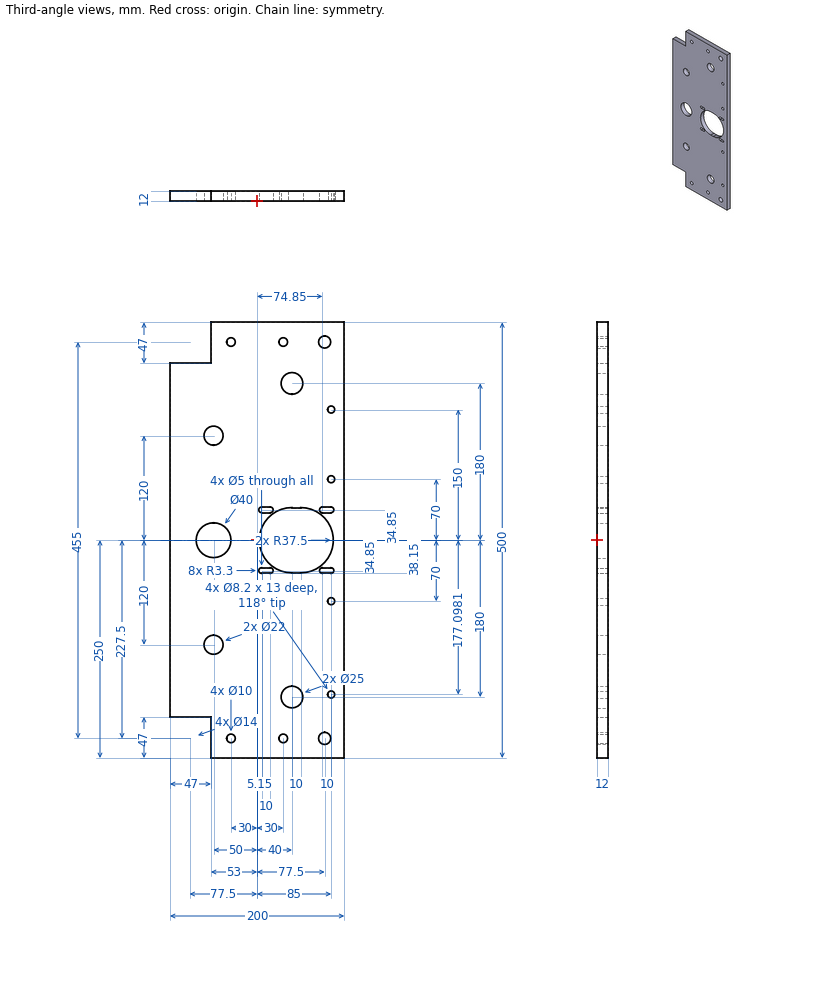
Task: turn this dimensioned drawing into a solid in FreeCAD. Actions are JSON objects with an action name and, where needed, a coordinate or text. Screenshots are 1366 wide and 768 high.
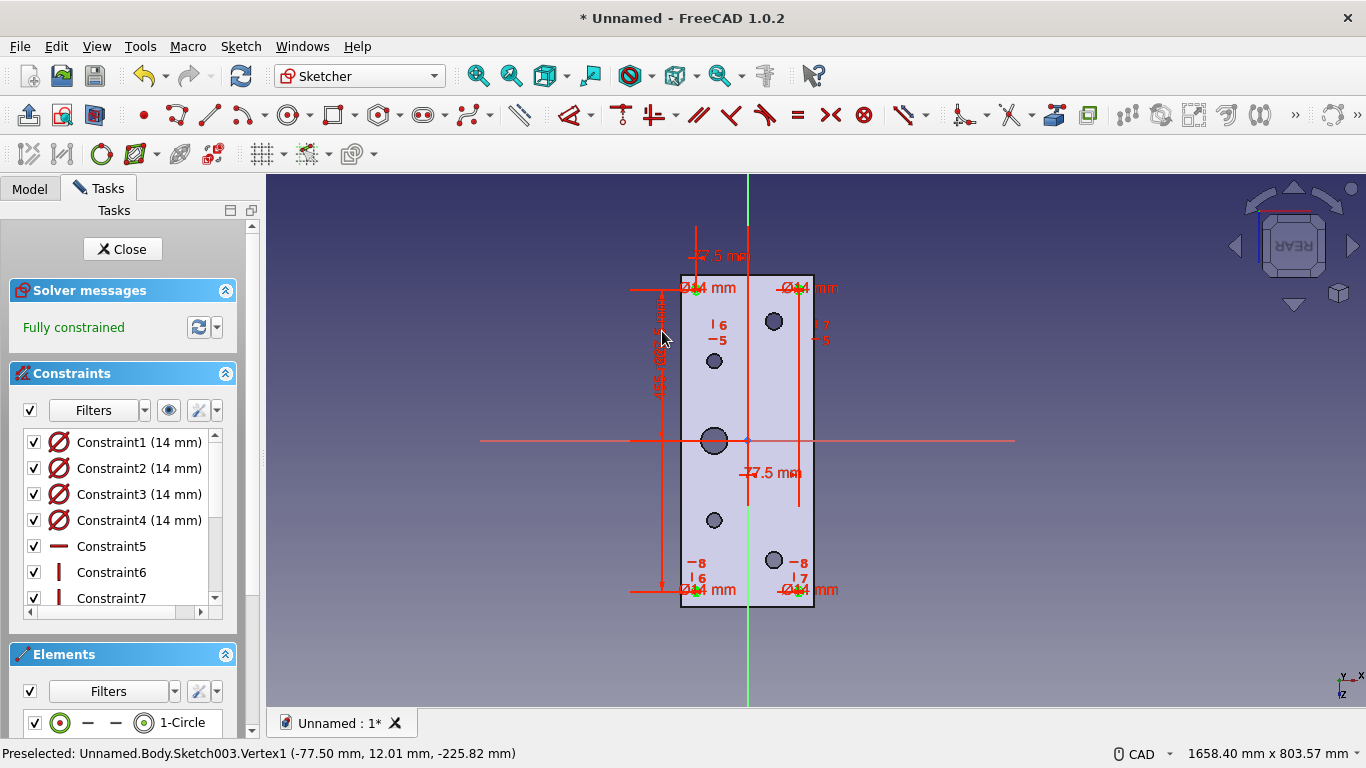
{"action": "left_click", "coordinate": [123, 249]}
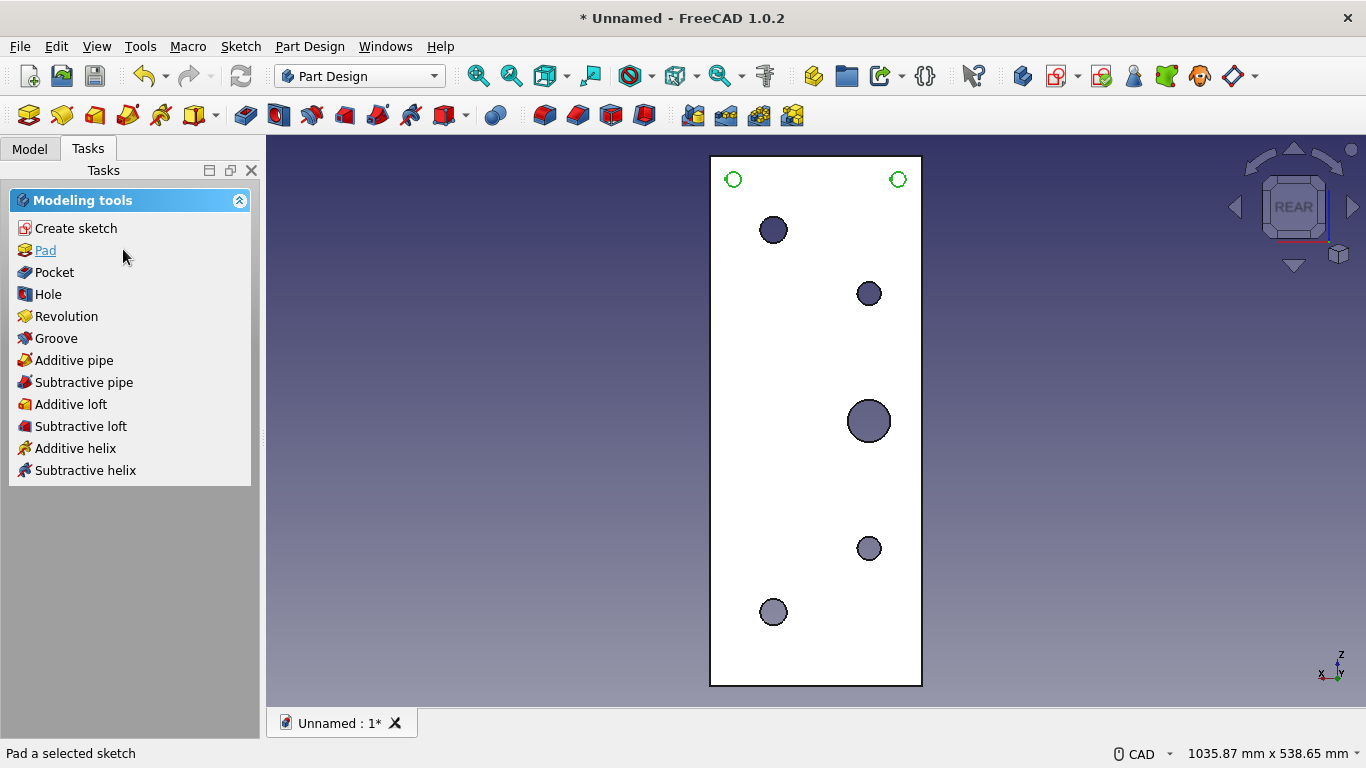
{"action": "left_click", "coordinate": [246, 116]}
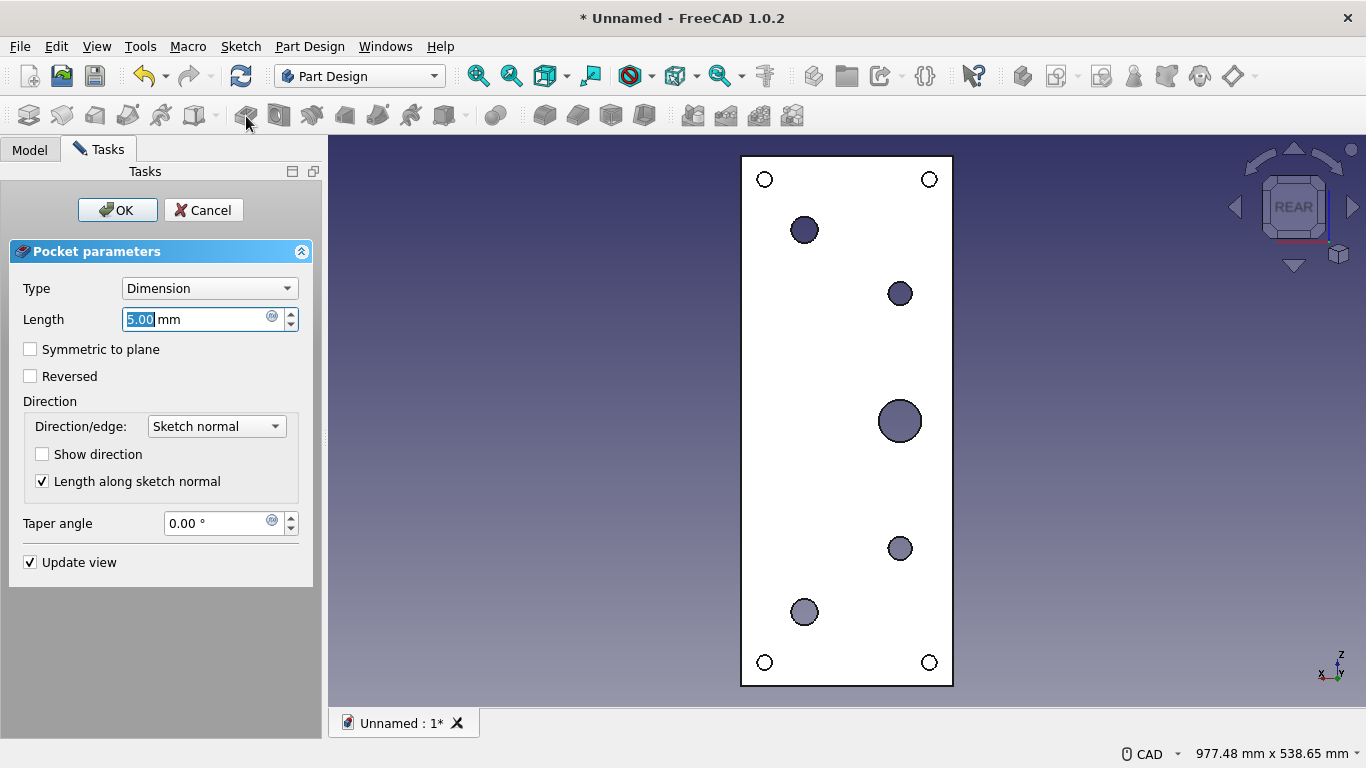
{"action": "type", "text": "12"}
{"action": "key", "text": "Tab"}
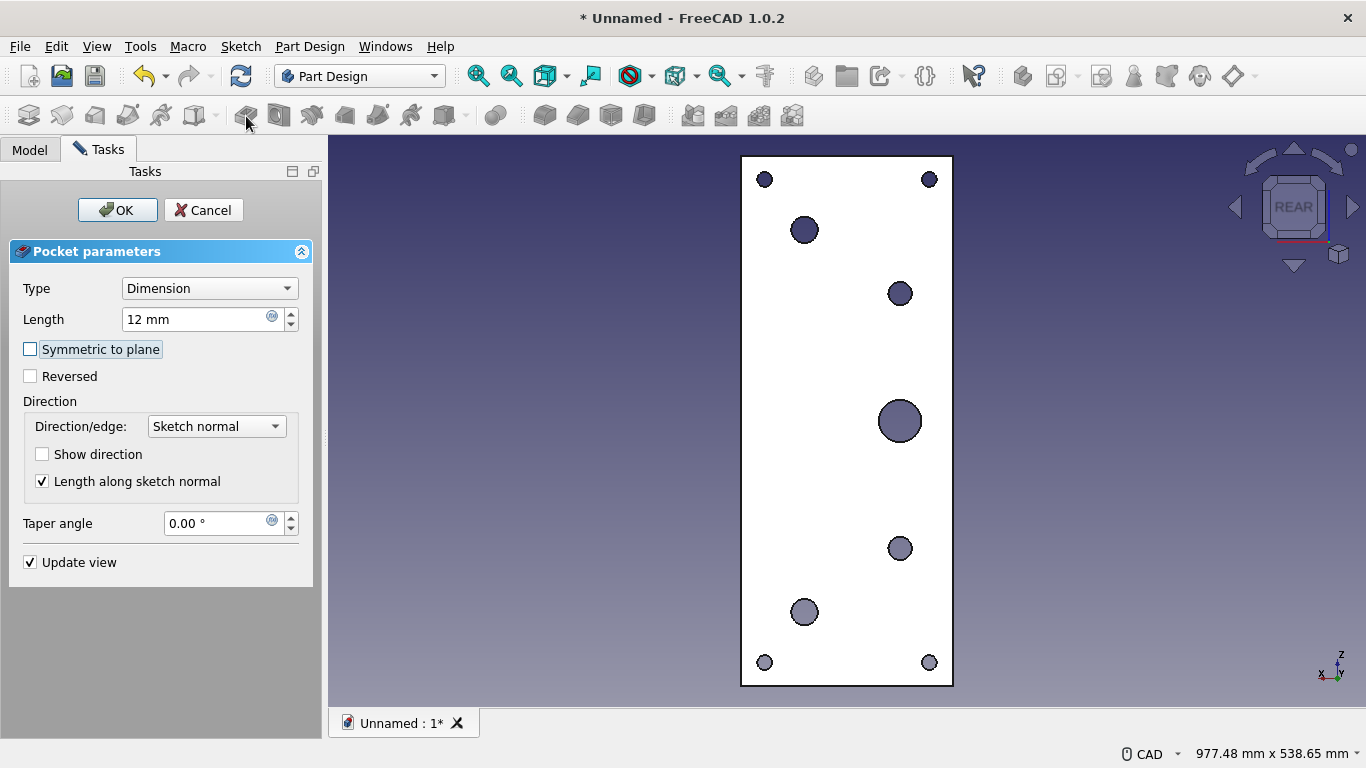
{"action": "left_click", "coordinate": [118, 210]}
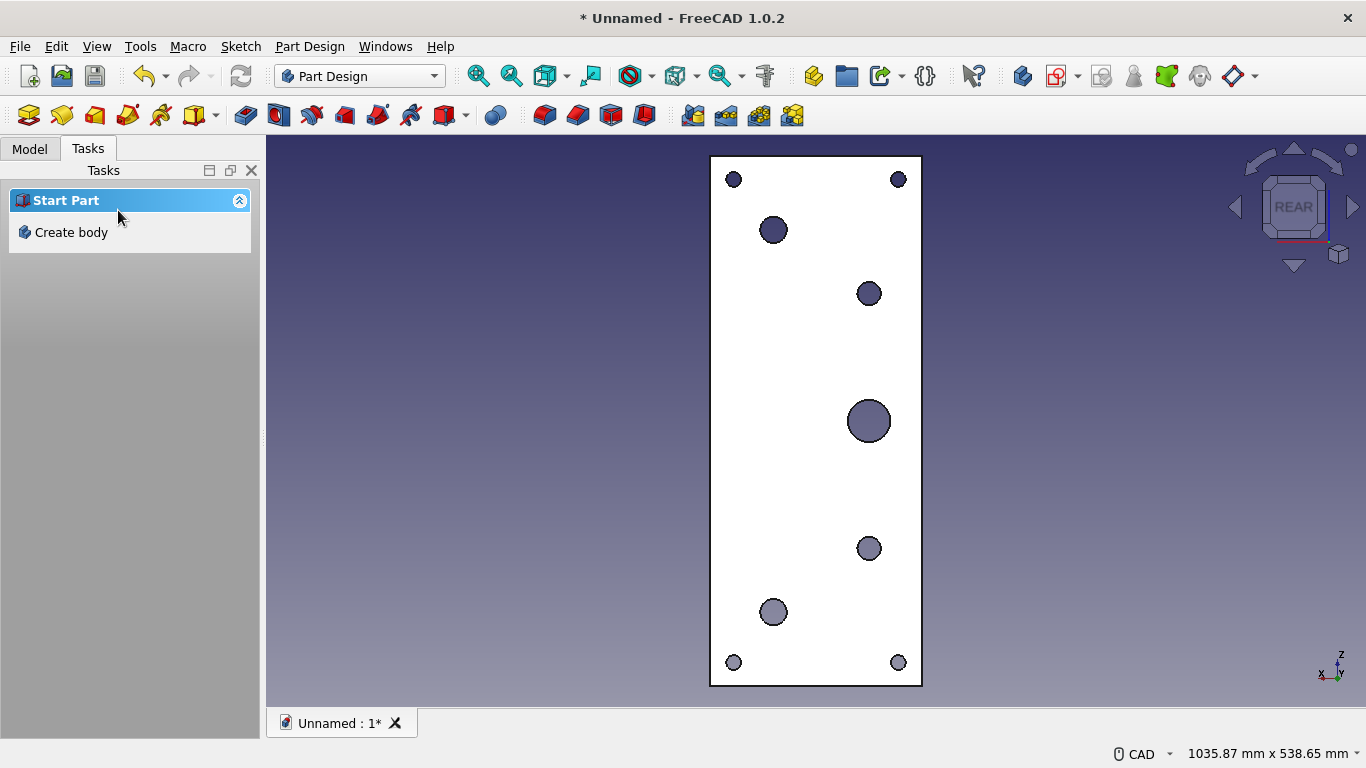
{"action": "left_click", "coordinate": [786, 344]}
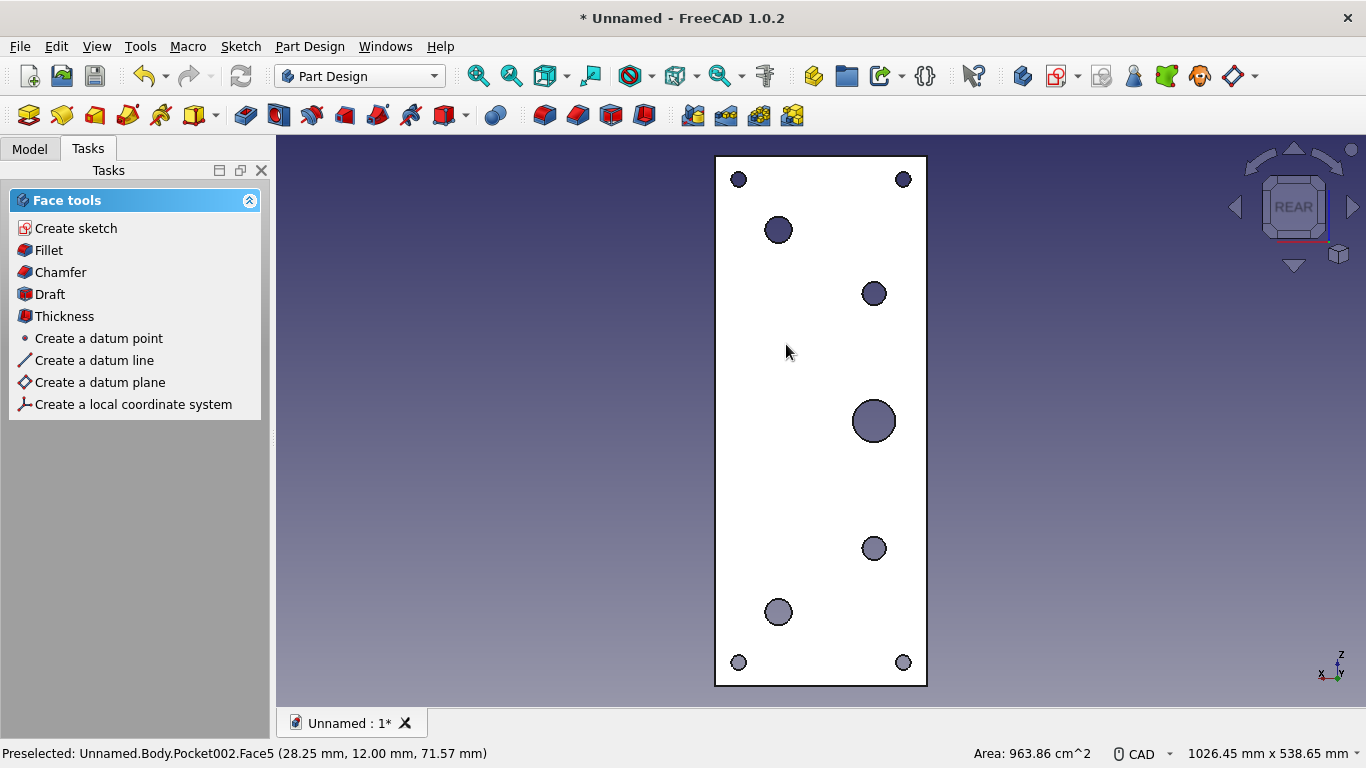
{"action": "left_click", "coordinate": [1056, 76]}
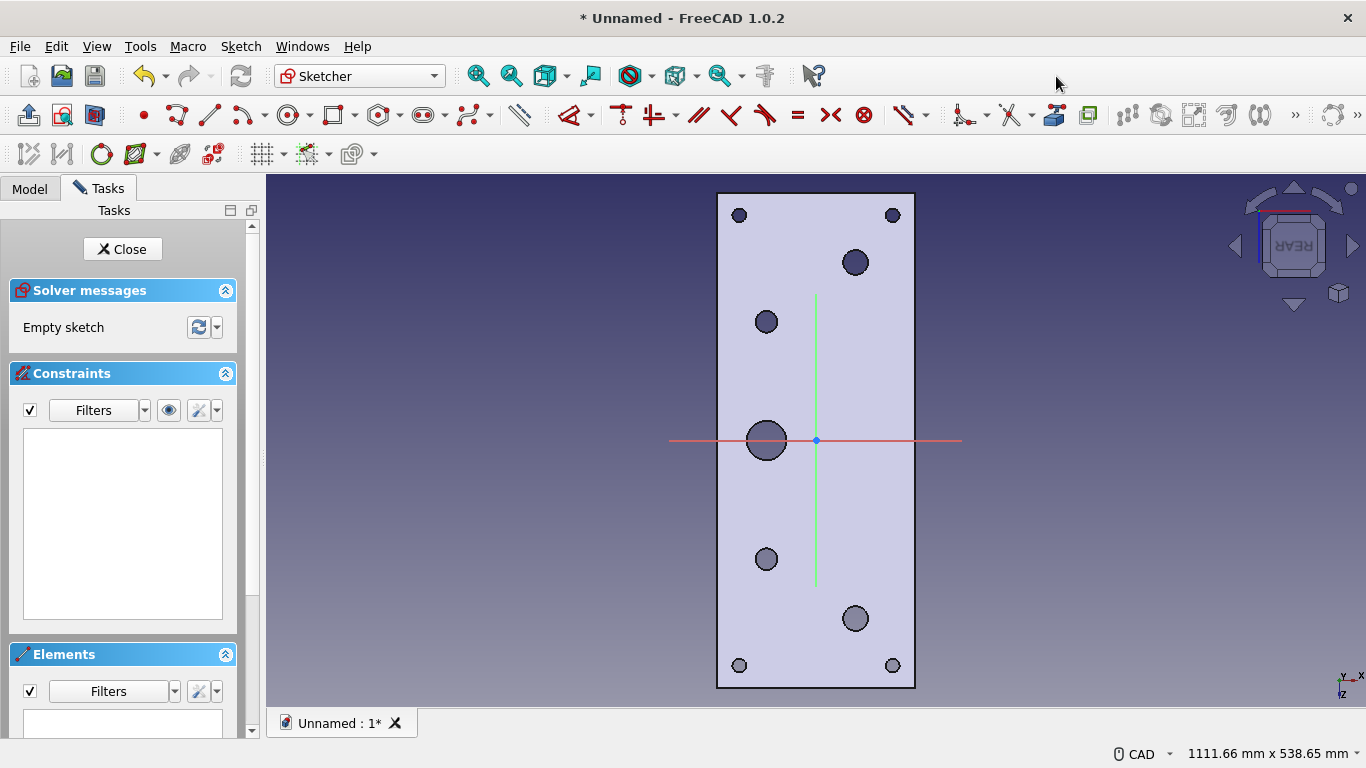
{"action": "left_click", "coordinate": [288, 116]}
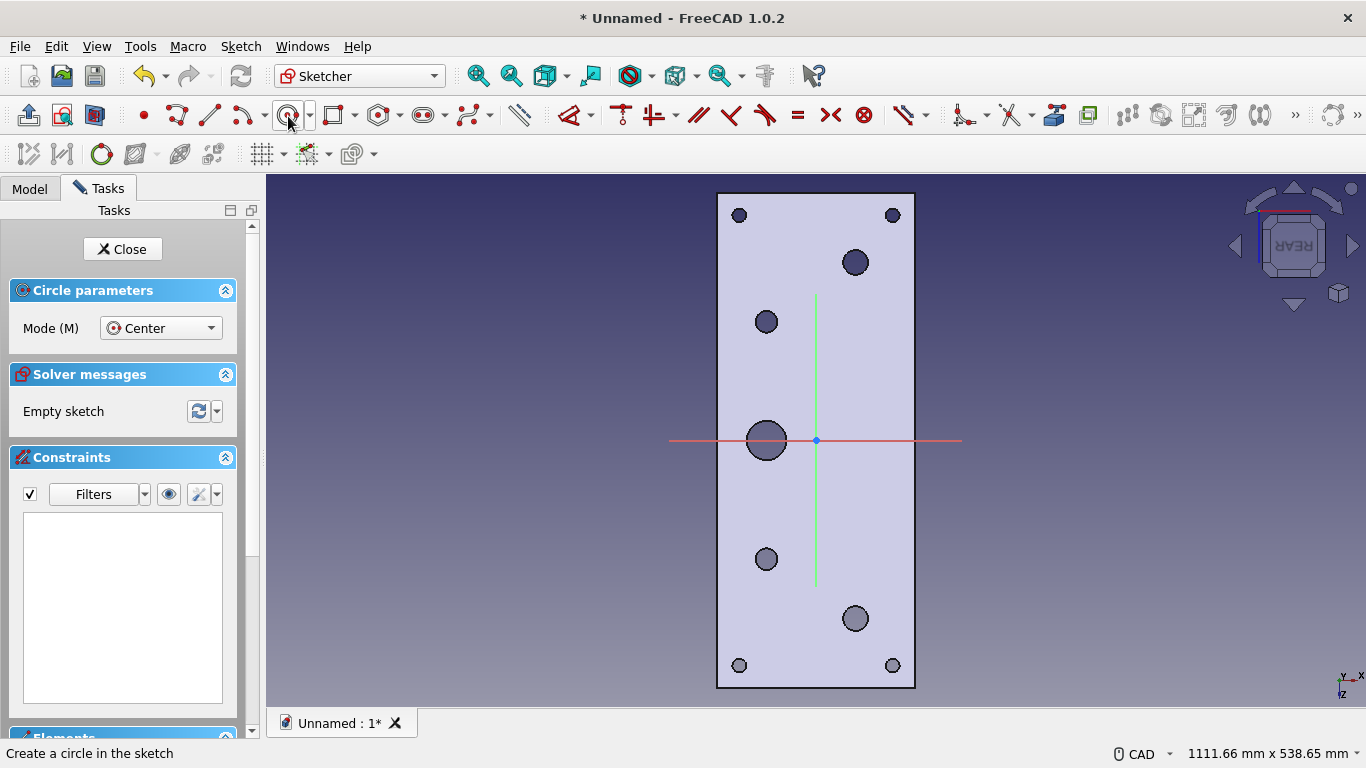
{"action": "scroll", "coordinate": [900, 265], "scroll_direction": "up", "scroll_amount": 9}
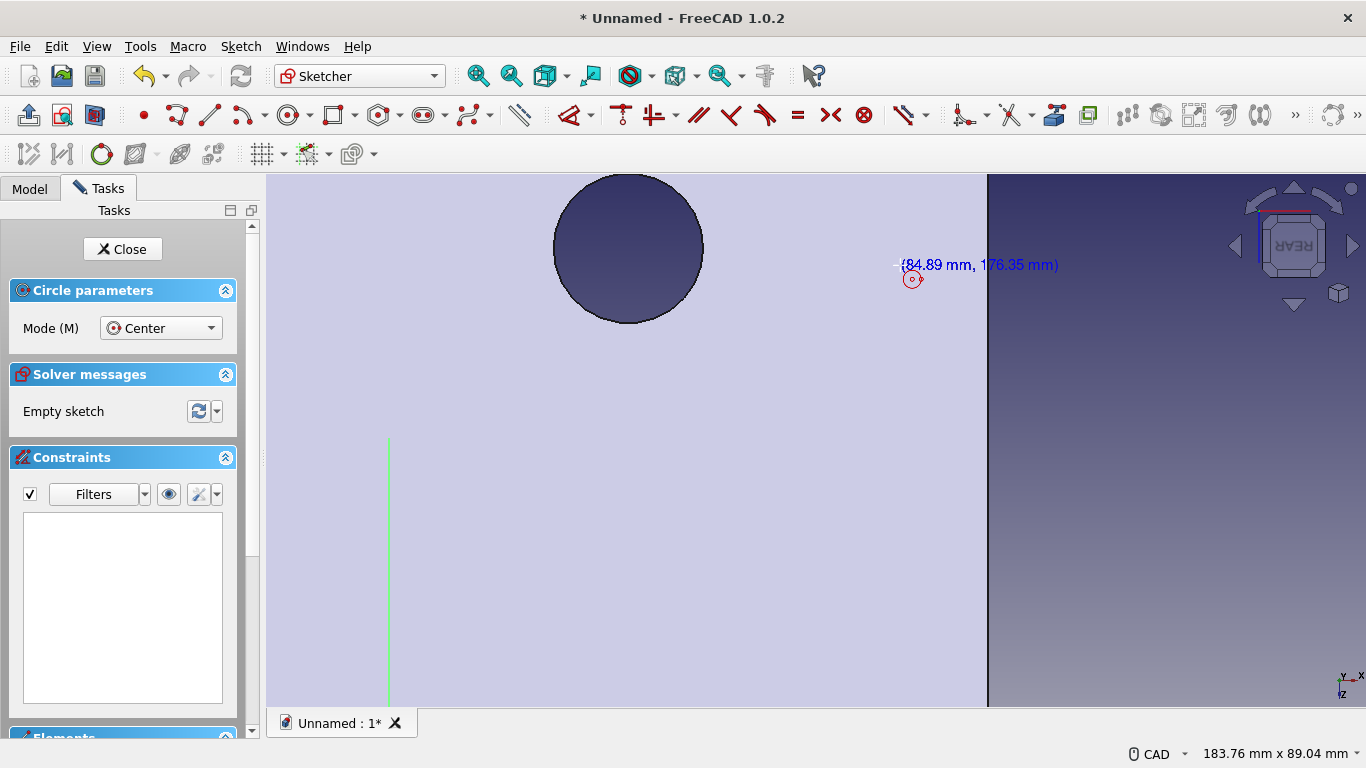
{"action": "scroll", "coordinate": [766, 281], "scroll_direction": "down", "scroll_amount": 9}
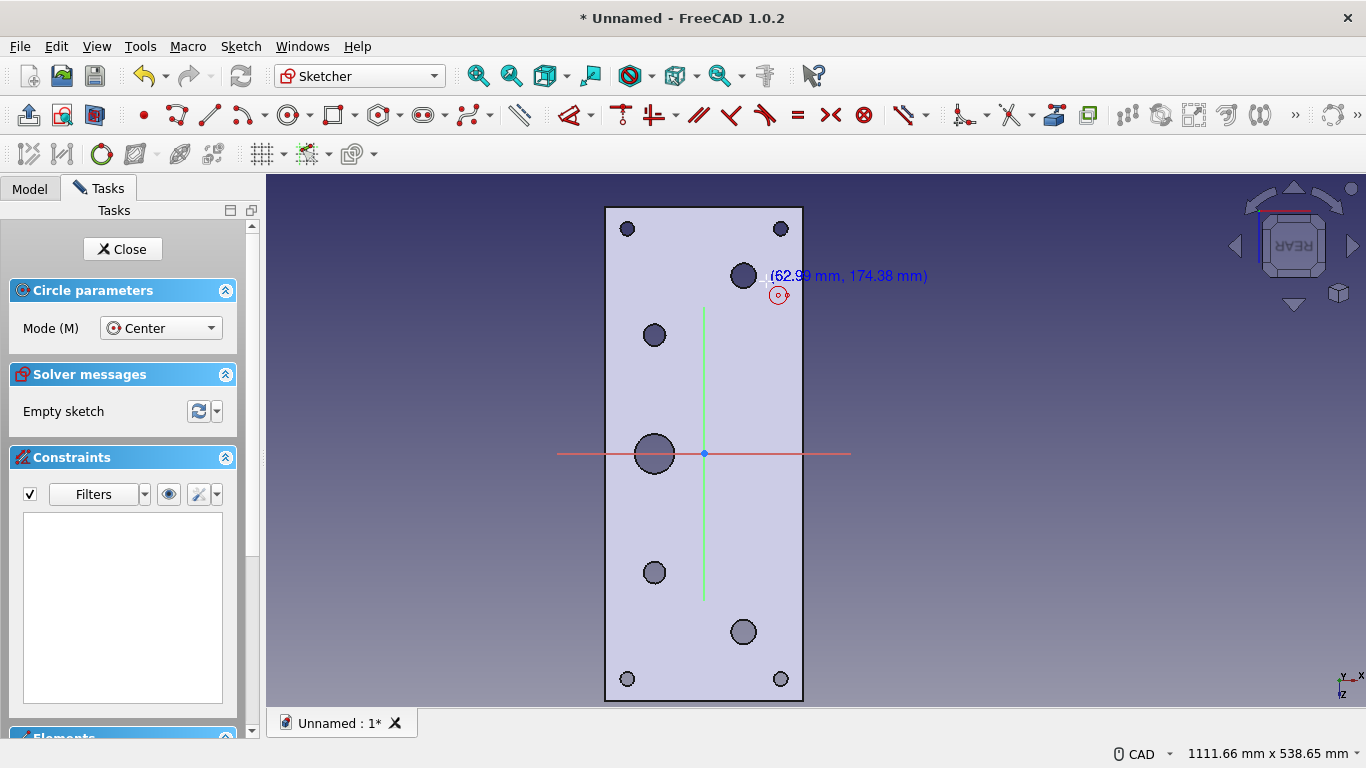
{"action": "left_click", "coordinate": [788, 279]}
{"action": "mouse_move", "coordinate": [791, 276]}